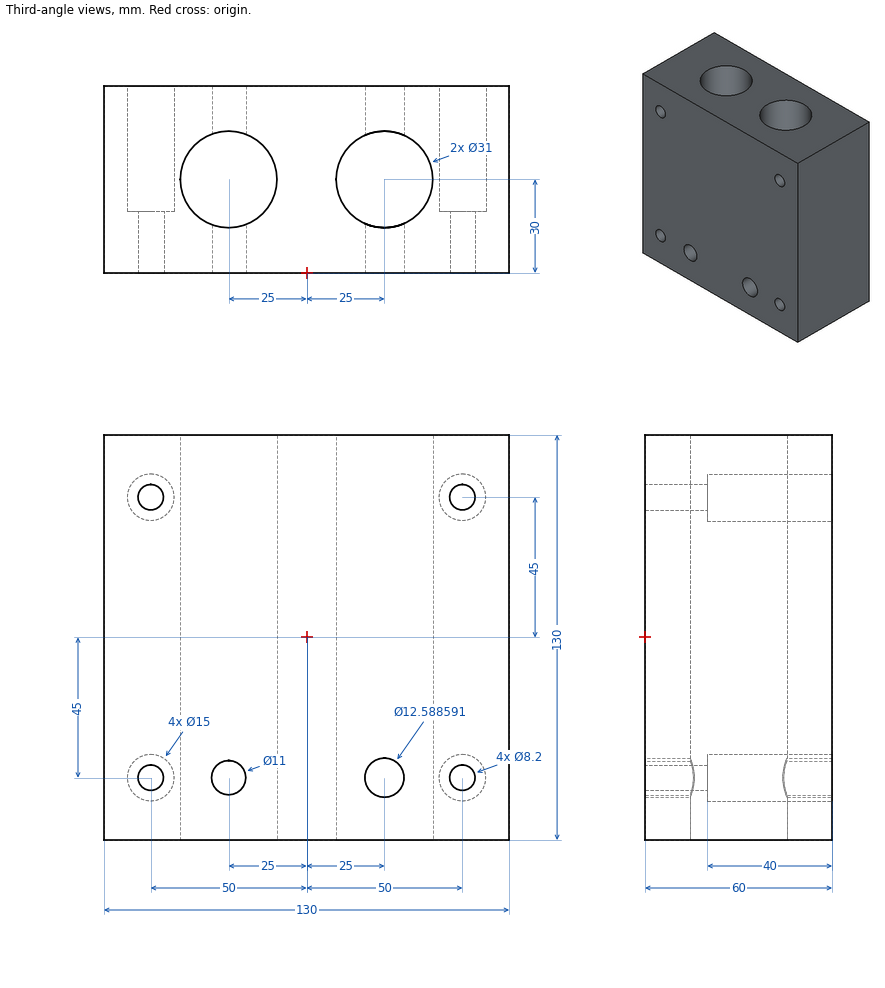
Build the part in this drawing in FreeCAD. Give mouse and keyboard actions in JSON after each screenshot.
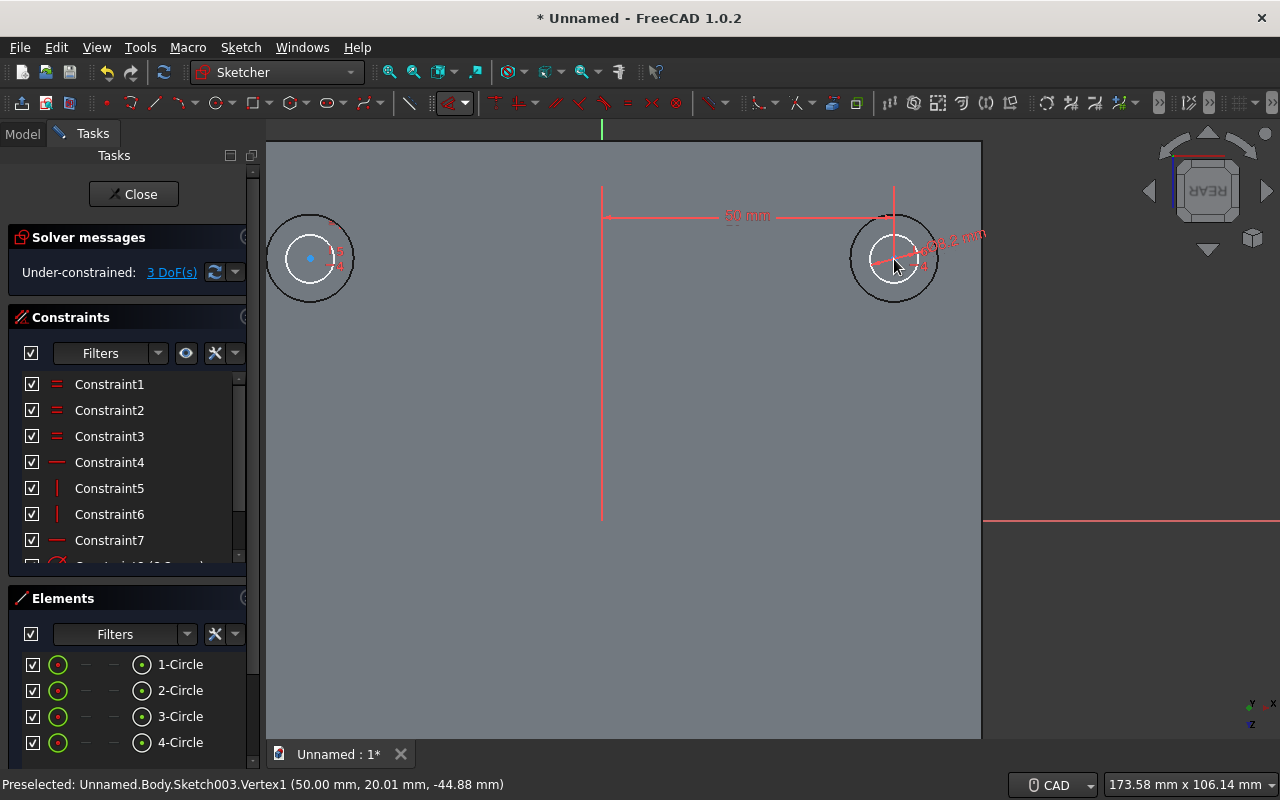
{"action": "left_click", "coordinate": [894, 259]}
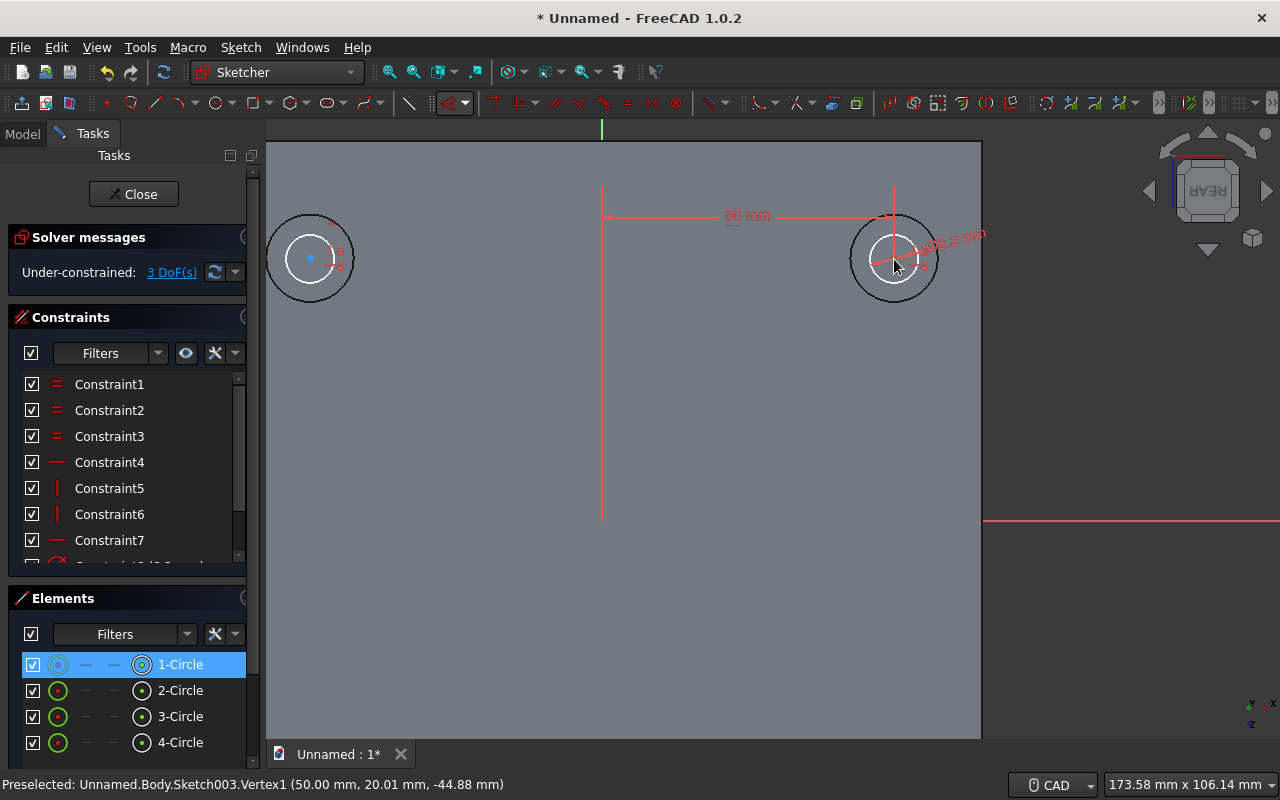
{"action": "key", "text": "i"}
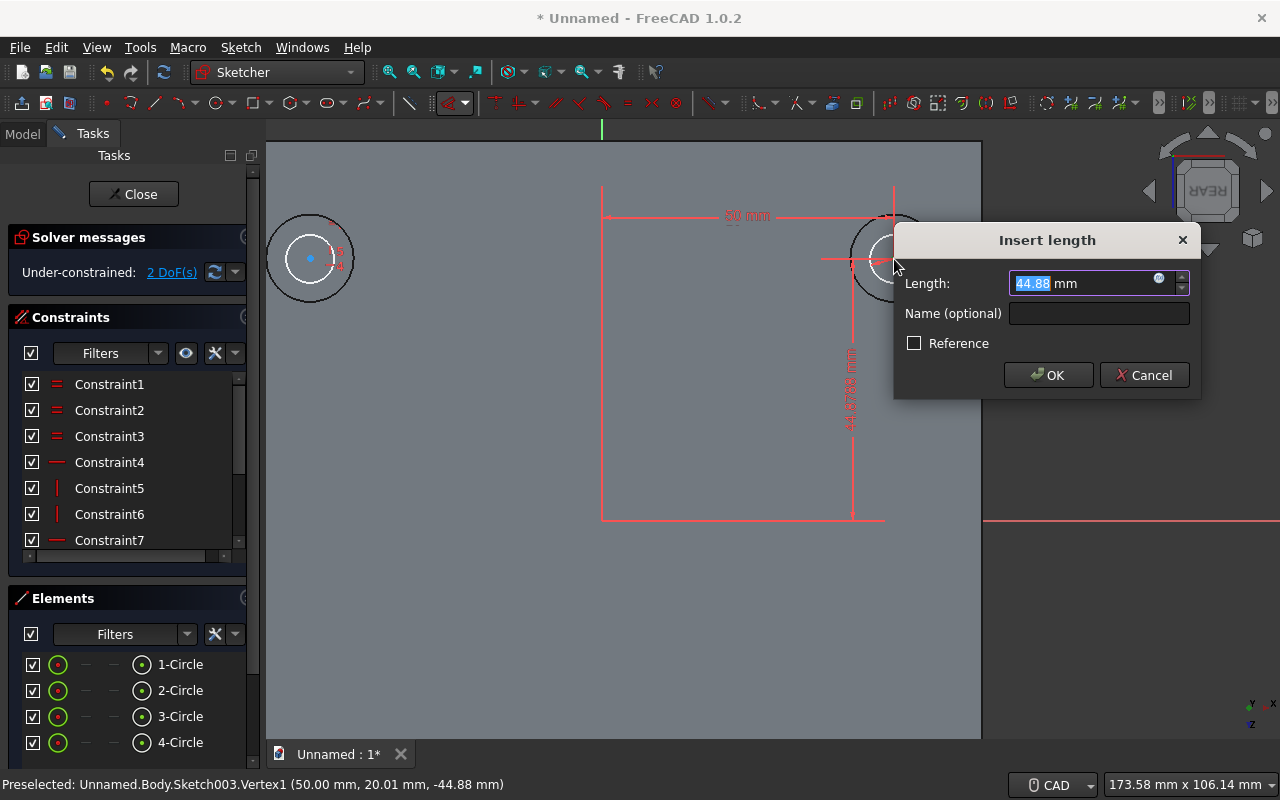
{"action": "type", "text": "45"}
{"action": "key", "text": "Return"}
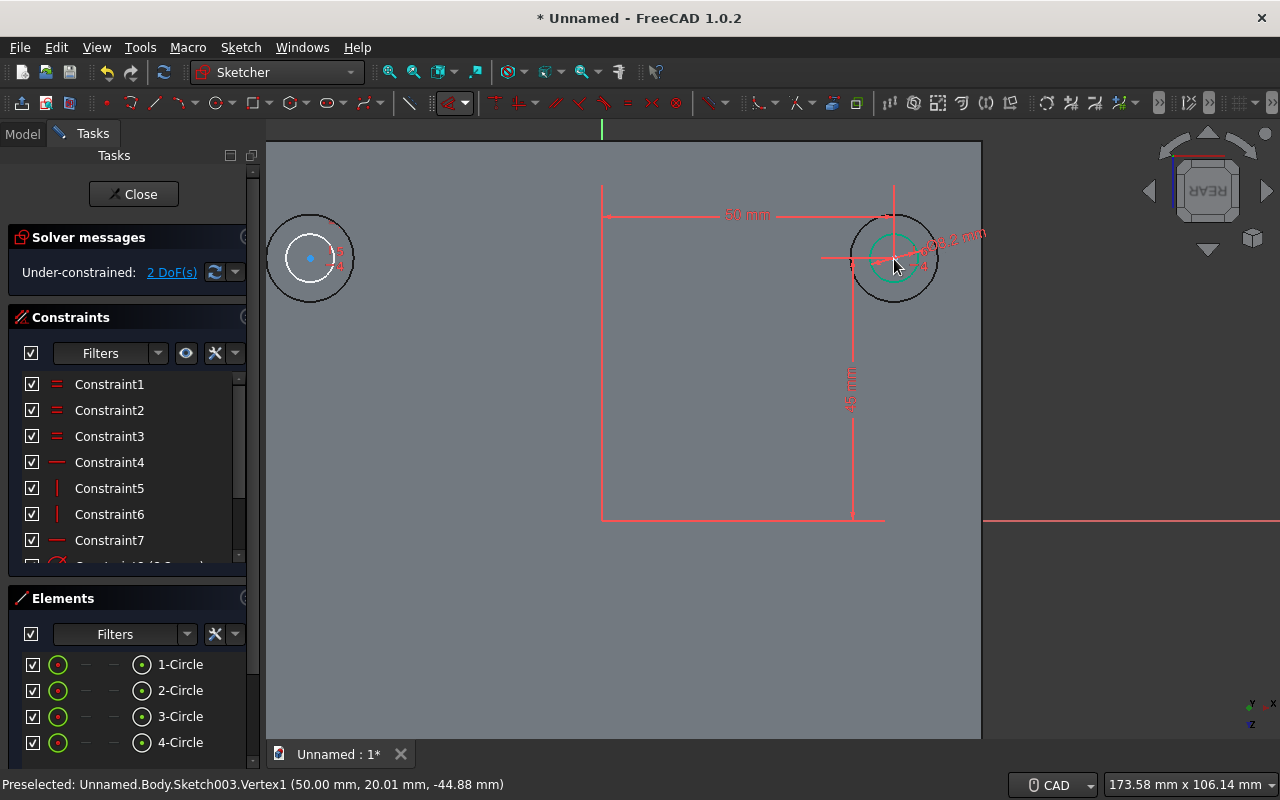
{"action": "left_click", "coordinate": [310, 258]}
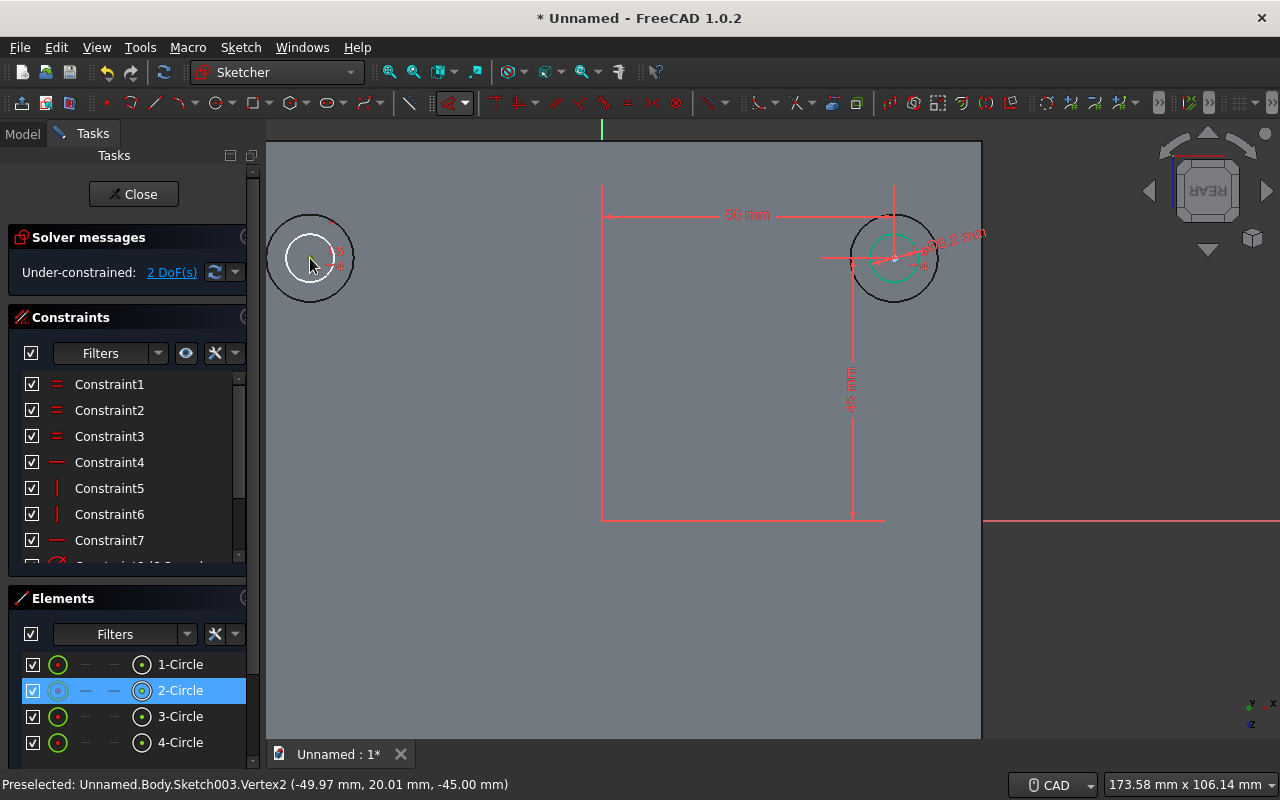
{"action": "key", "text": "l"}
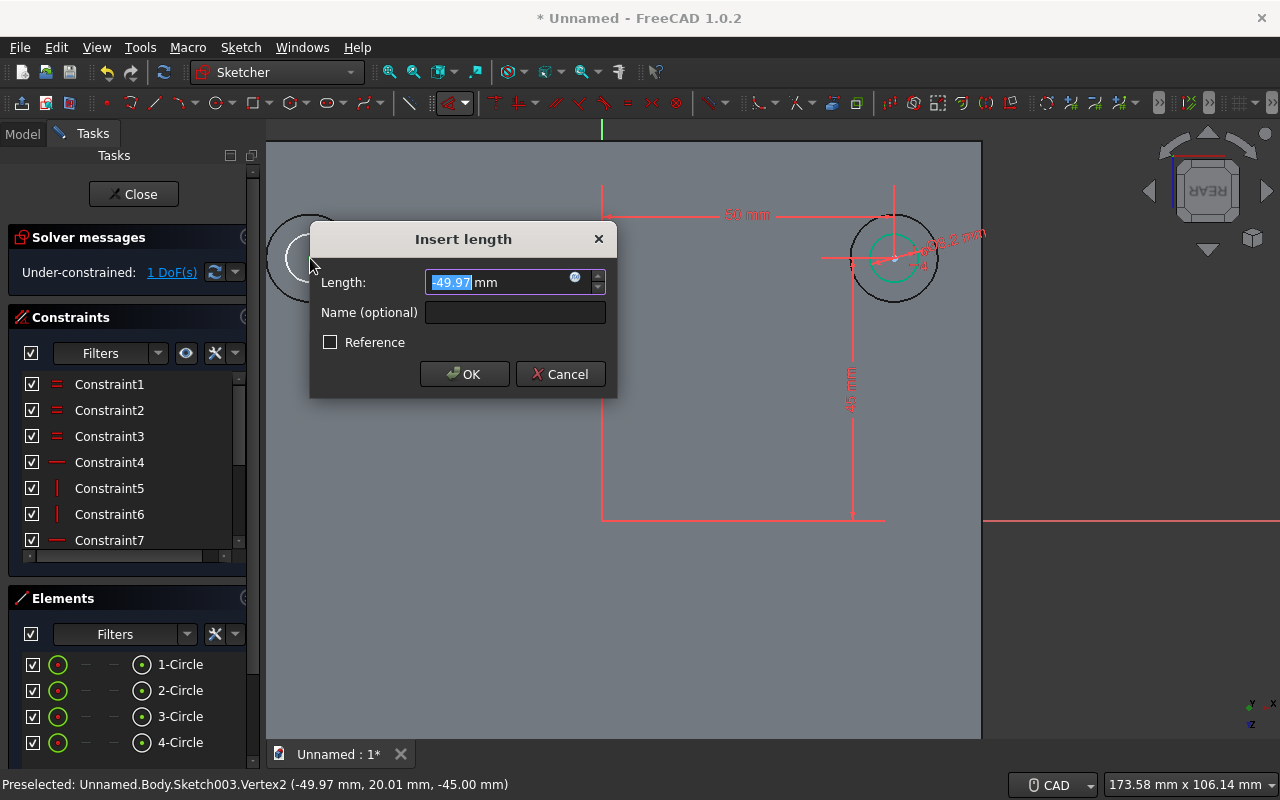
{"action": "type", "text": "-50"}
{"action": "key", "text": "Return"}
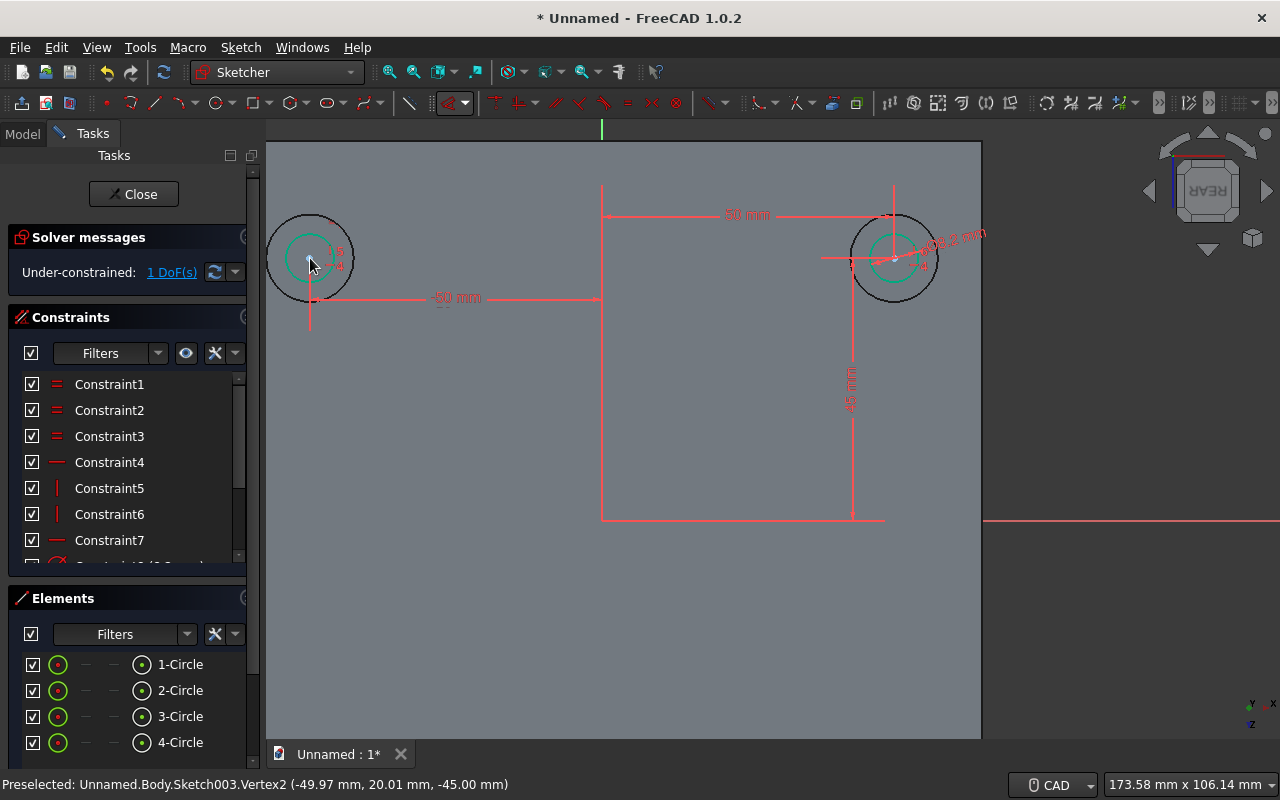
{"action": "scroll", "coordinate": [913, 242], "scroll_direction": "down", "scroll_amount": 2}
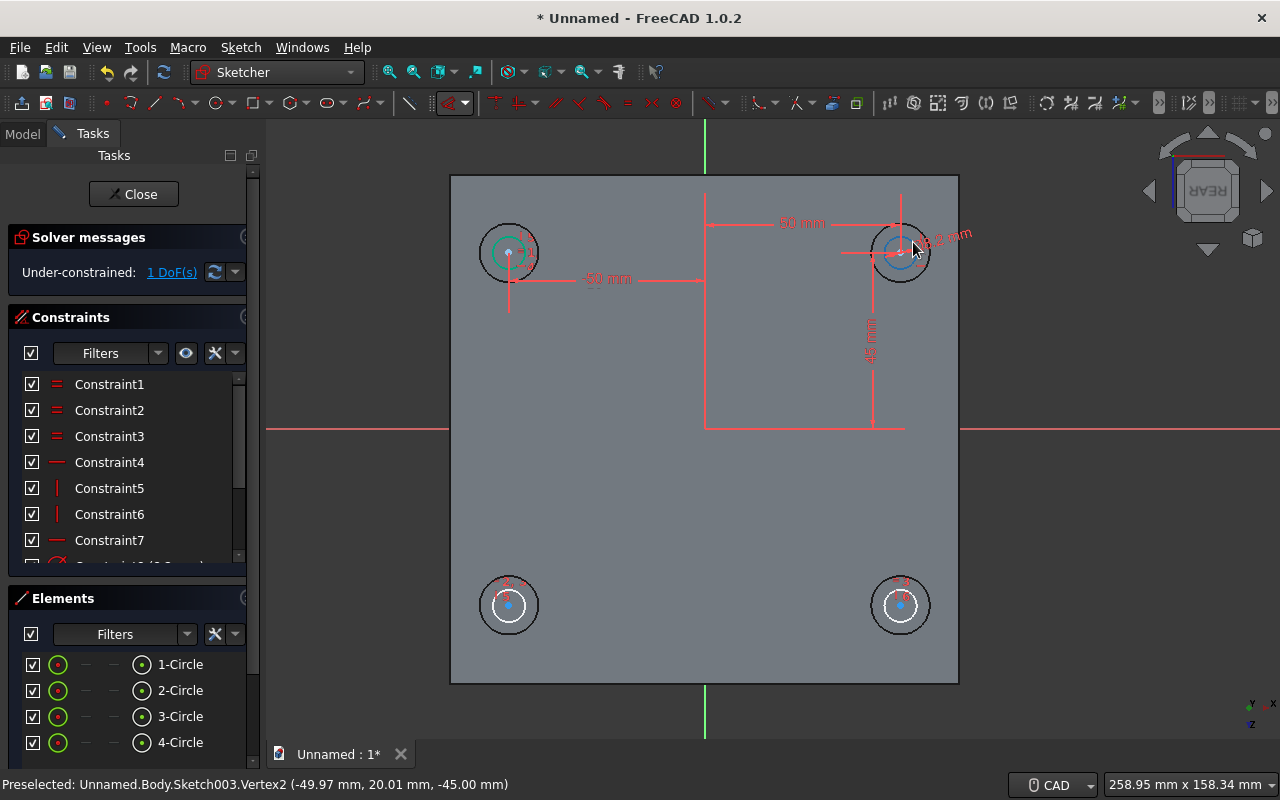
{"action": "left_click", "coordinate": [509, 606]}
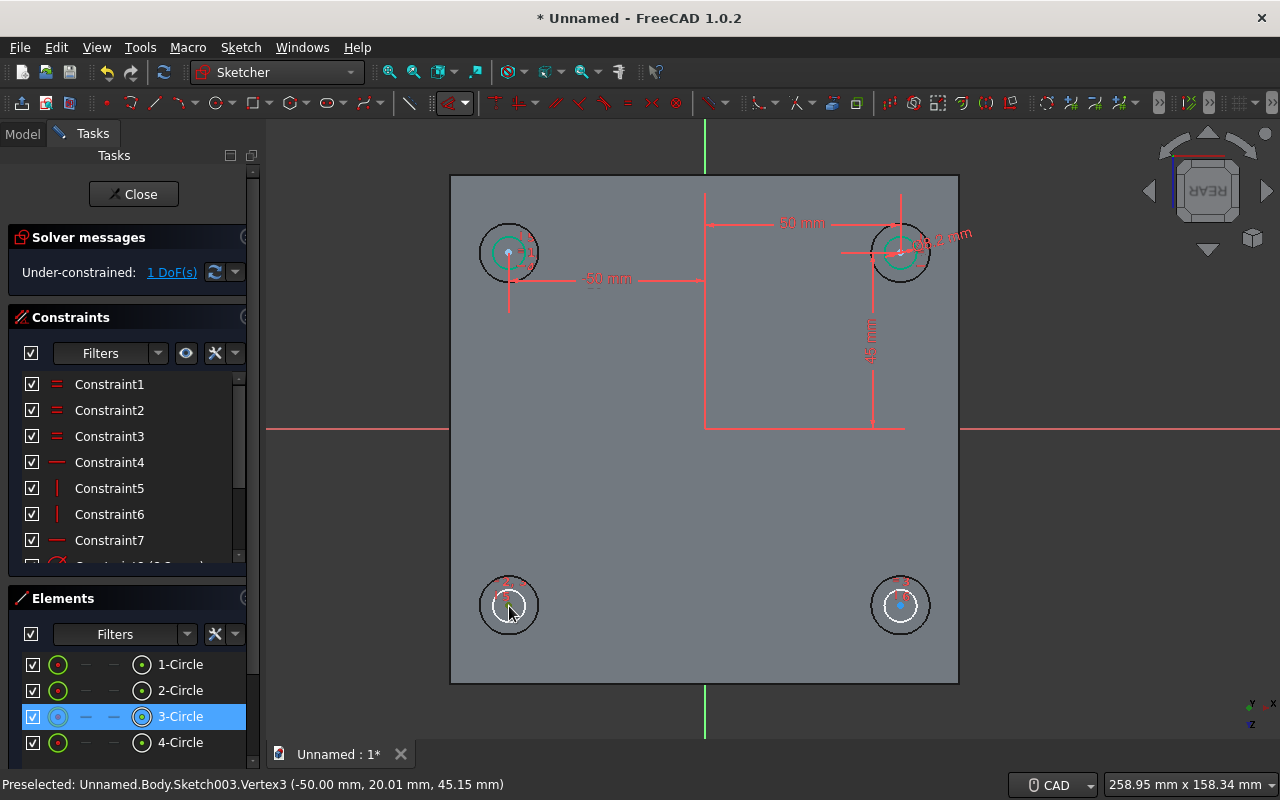
{"action": "key", "text": "i"}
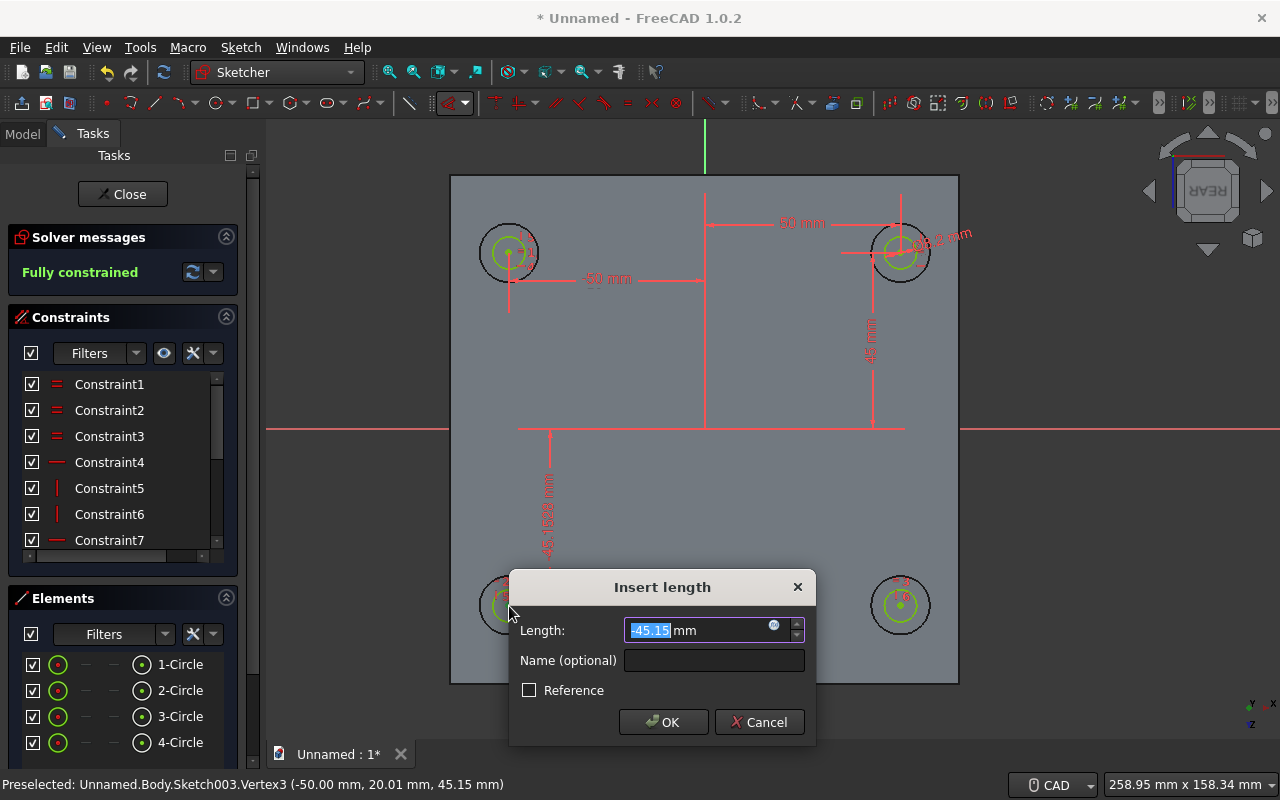
{"action": "type", "text": "-45"}
{"action": "key", "text": "Return"}